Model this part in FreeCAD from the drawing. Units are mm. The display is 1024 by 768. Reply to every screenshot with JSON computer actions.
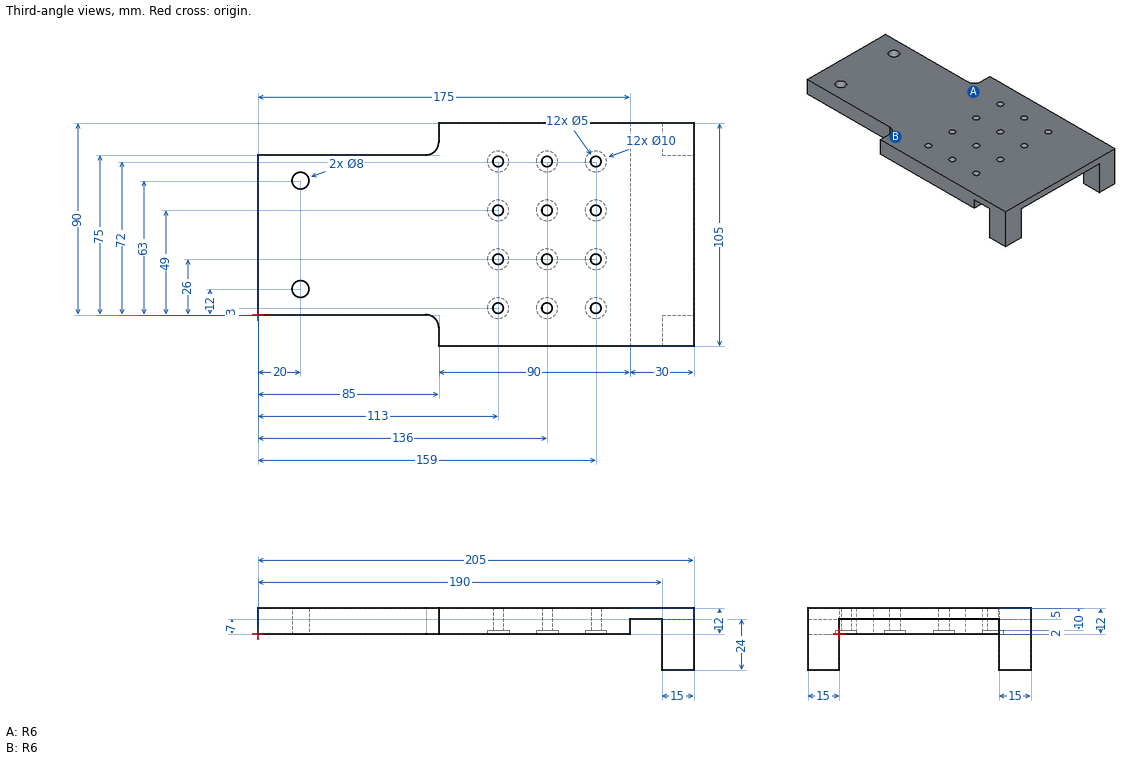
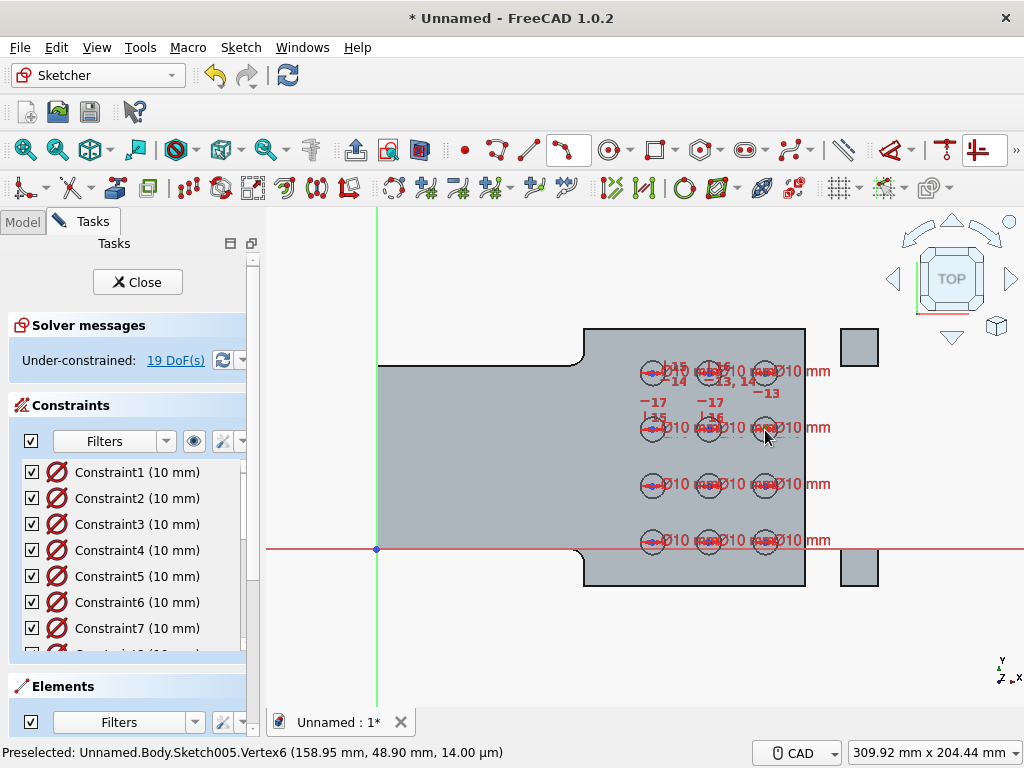
{"action": "left_click", "coordinate": [1002, 150]}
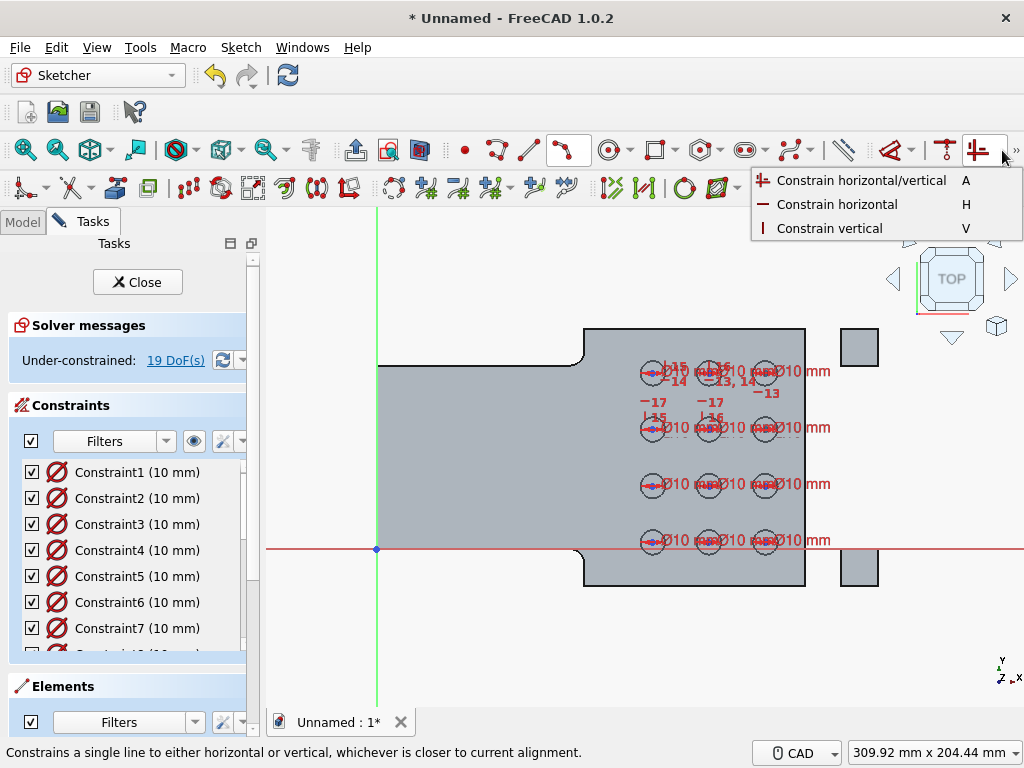
{"action": "left_click", "coordinate": [887, 228]}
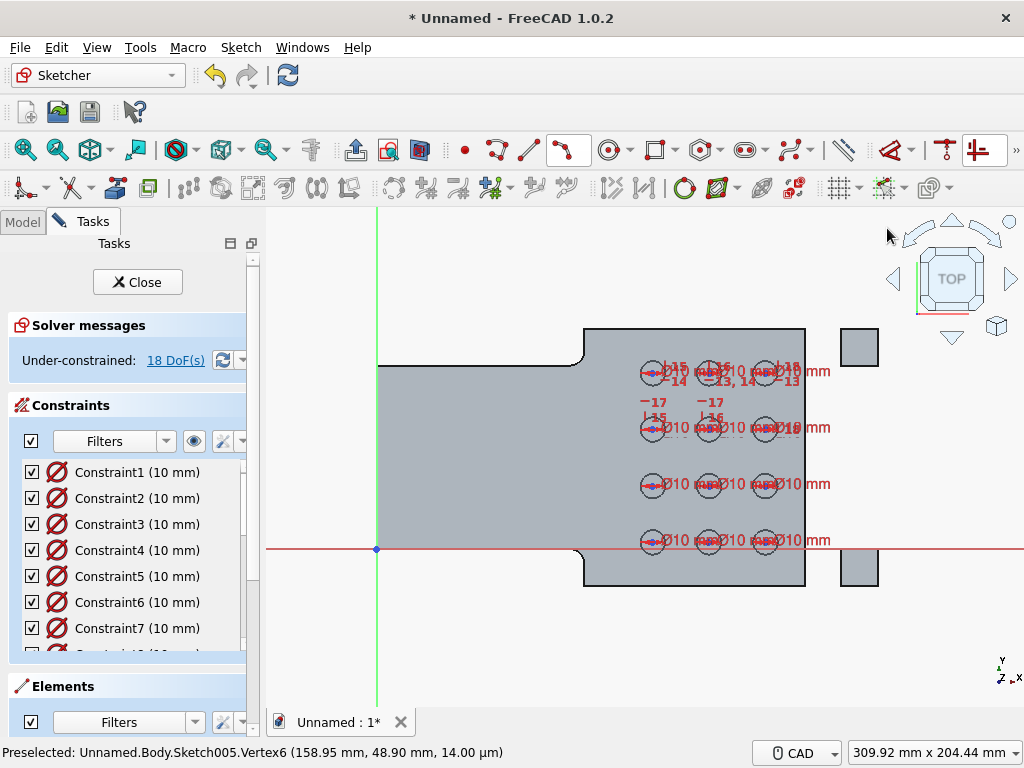
{"action": "left_click", "coordinate": [709, 430]}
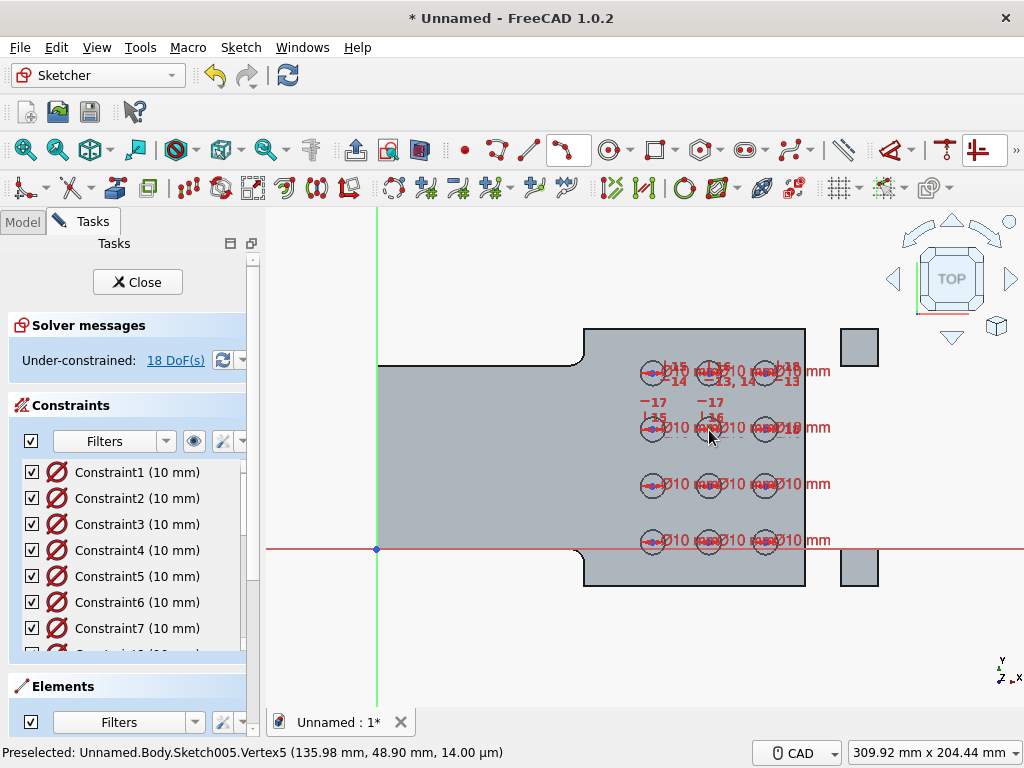
{"action": "left_click", "coordinate": [765, 430]}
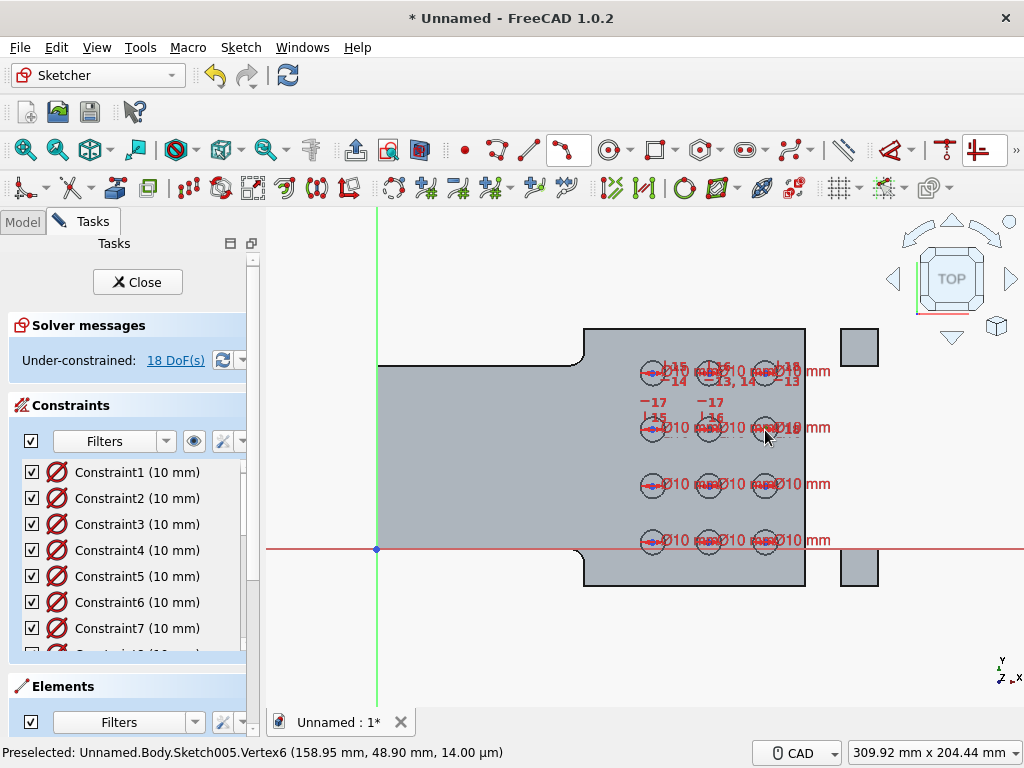
{"action": "key", "text": "h"}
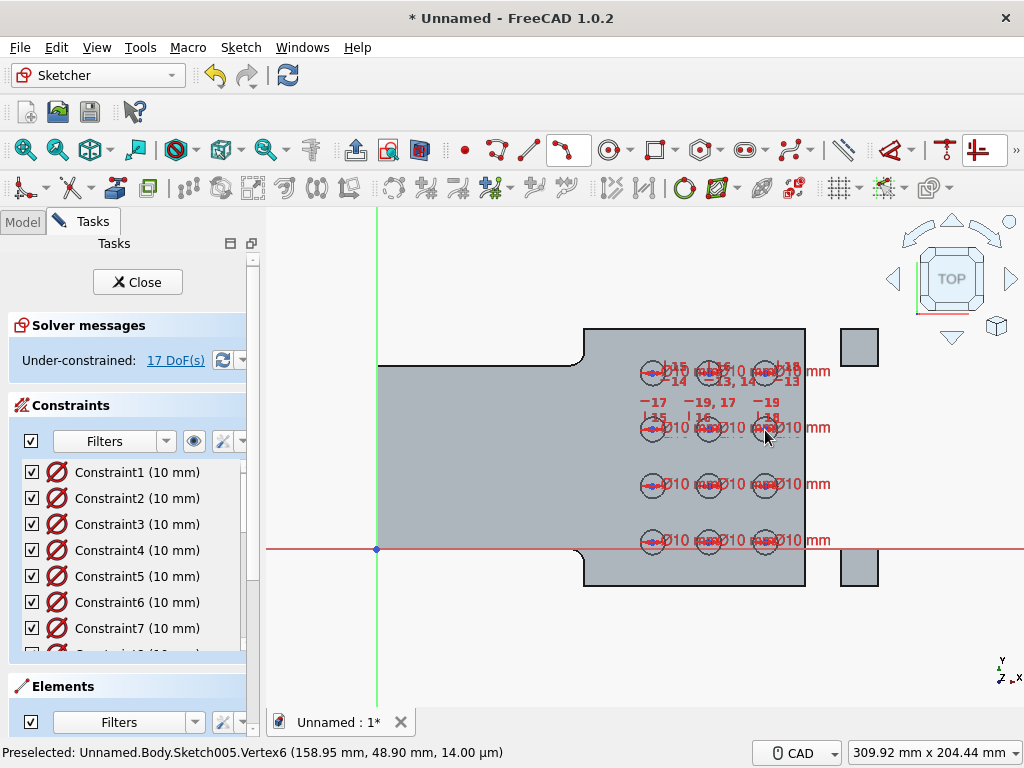
{"action": "left_click", "coordinate": [765, 430]}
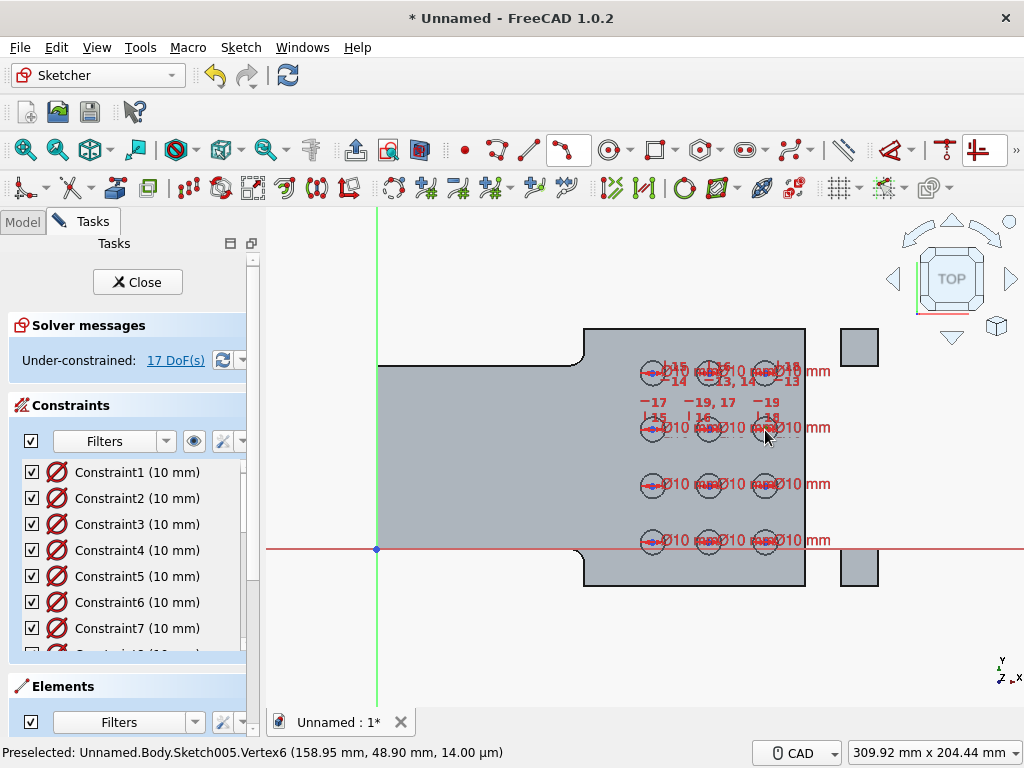
{"action": "left_click", "coordinate": [765, 486]}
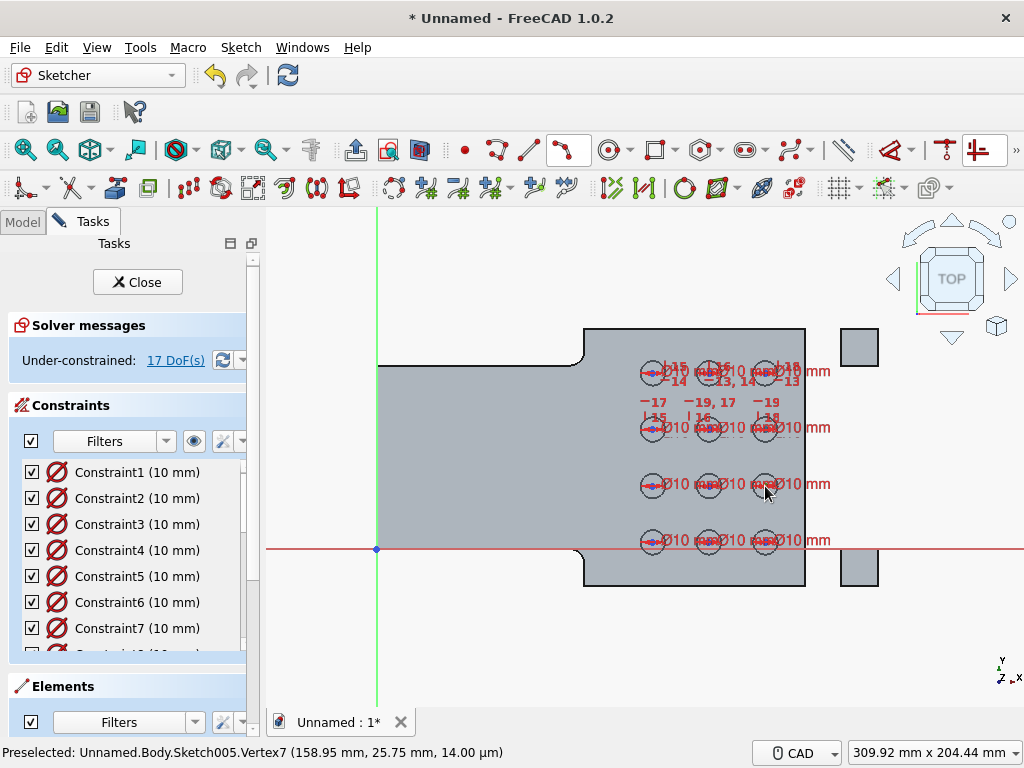
{"action": "left_click", "coordinate": [1002, 150]}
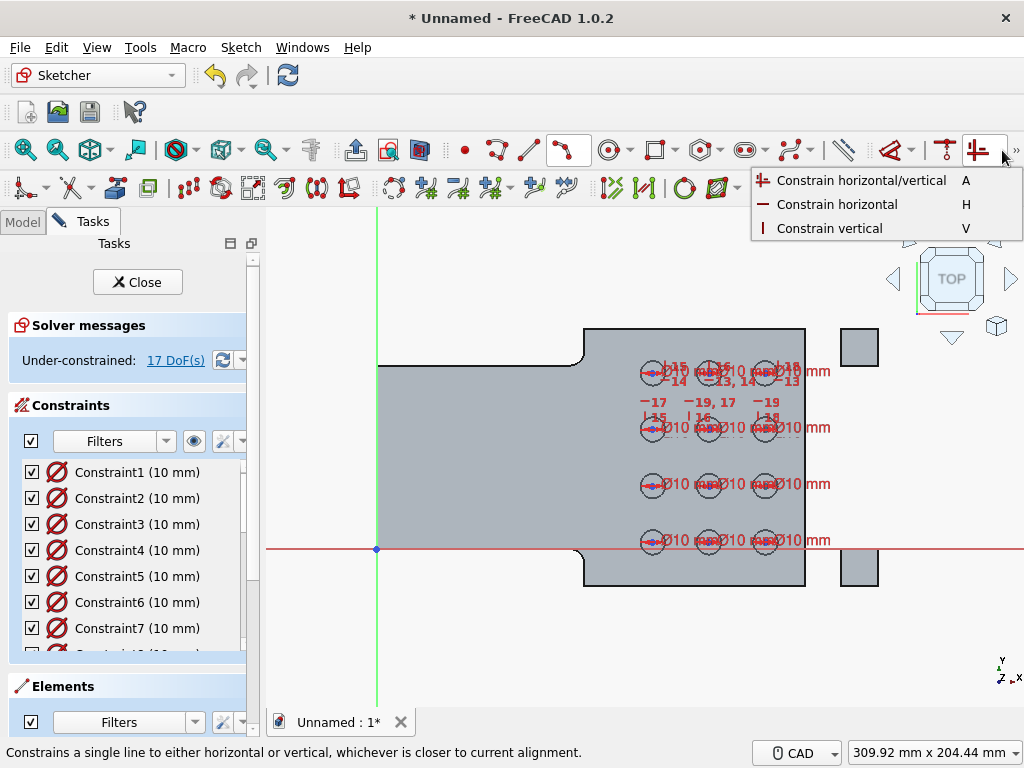
{"action": "left_click", "coordinate": [887, 228]}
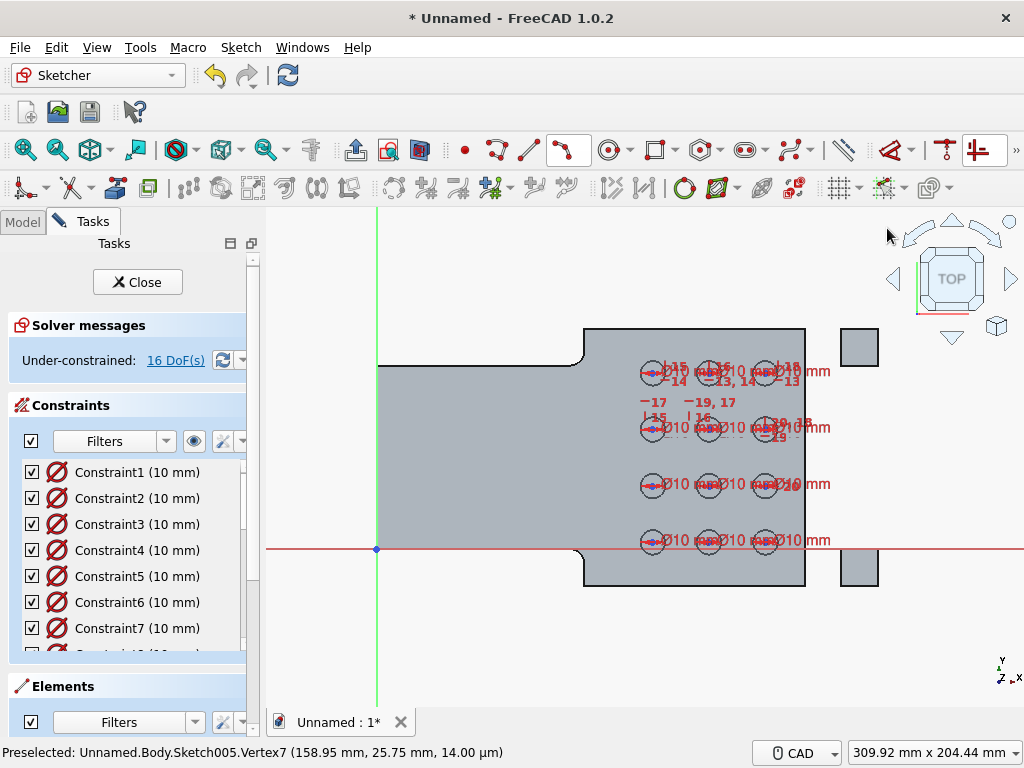
{"action": "left_click", "coordinate": [709, 430]}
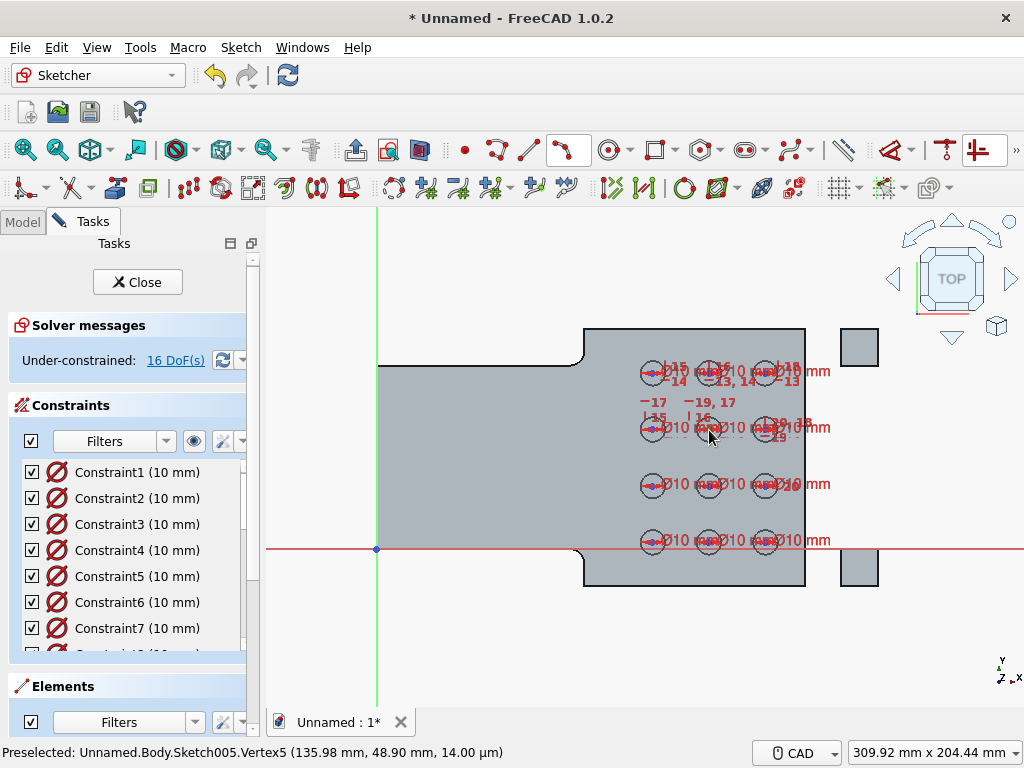
{"action": "left_click", "coordinate": [709, 486]}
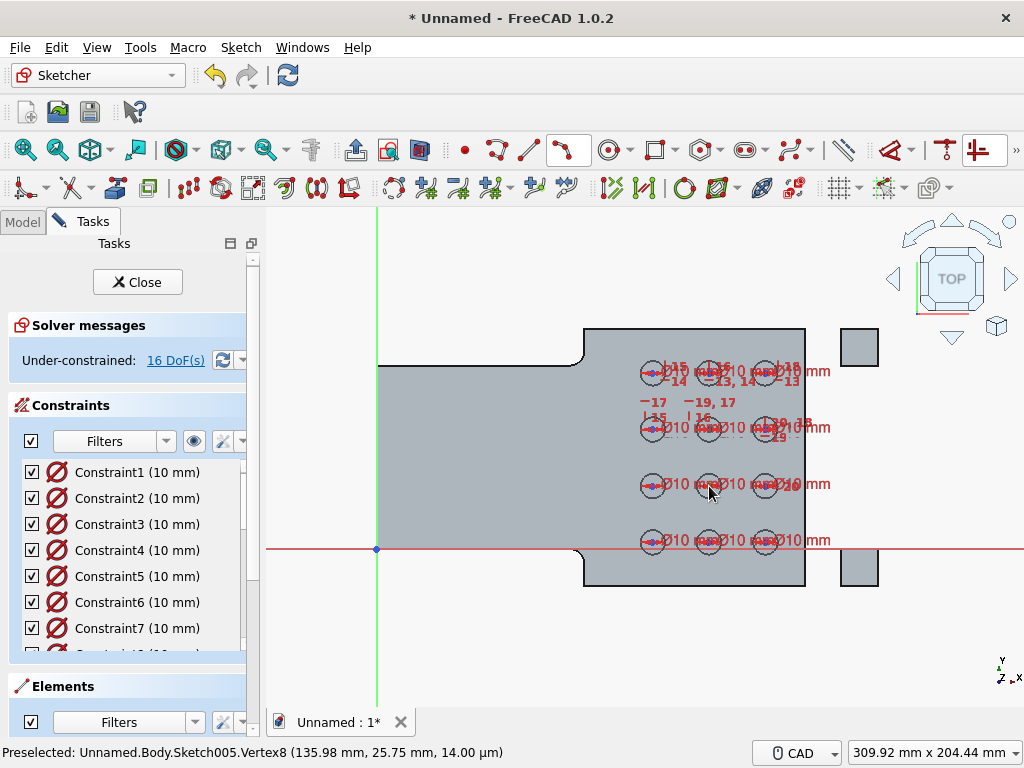
{"action": "key", "text": "v"}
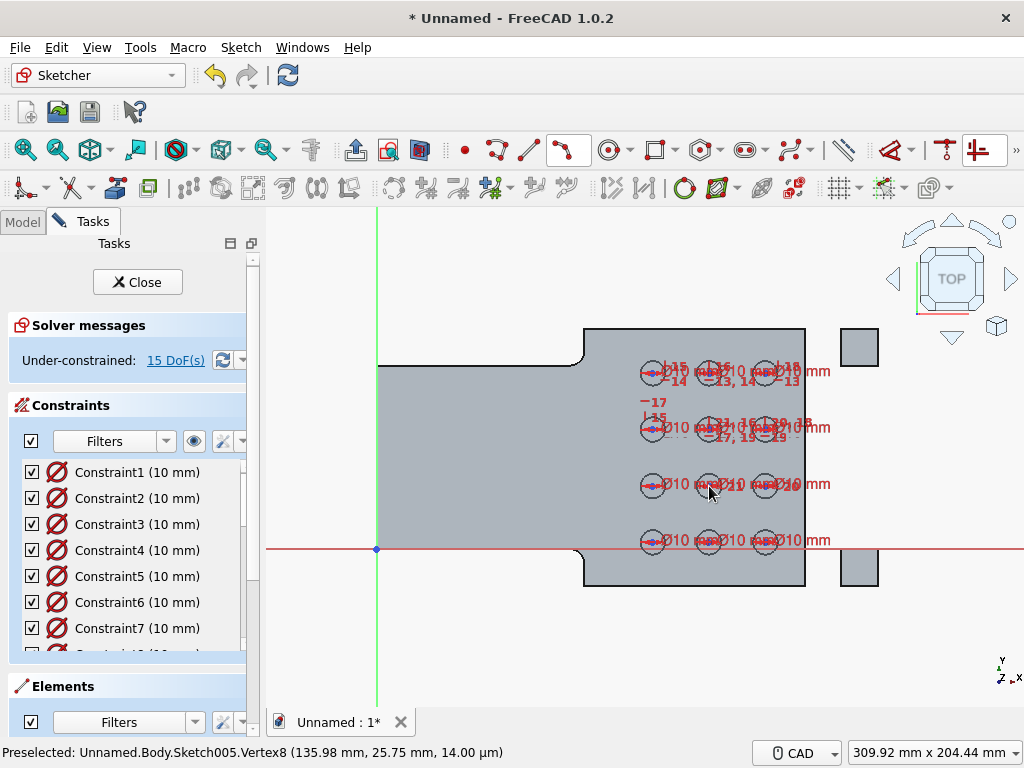
{"action": "left_click", "coordinate": [765, 486]}